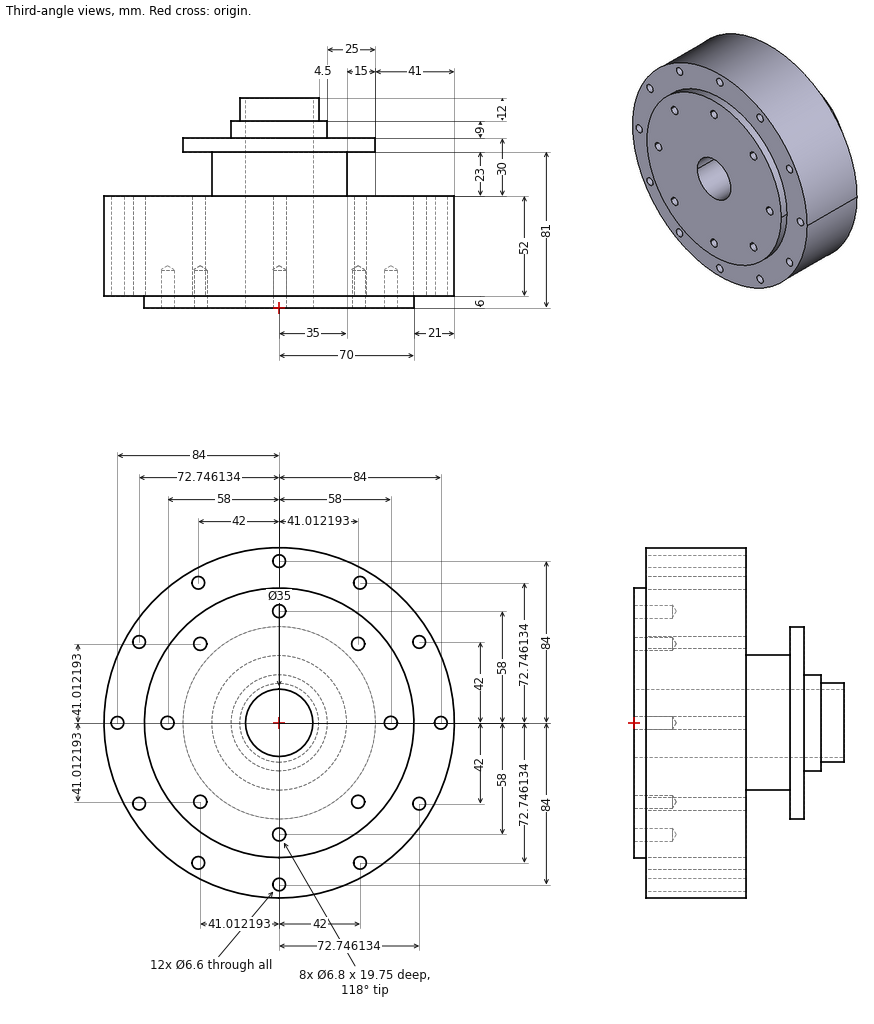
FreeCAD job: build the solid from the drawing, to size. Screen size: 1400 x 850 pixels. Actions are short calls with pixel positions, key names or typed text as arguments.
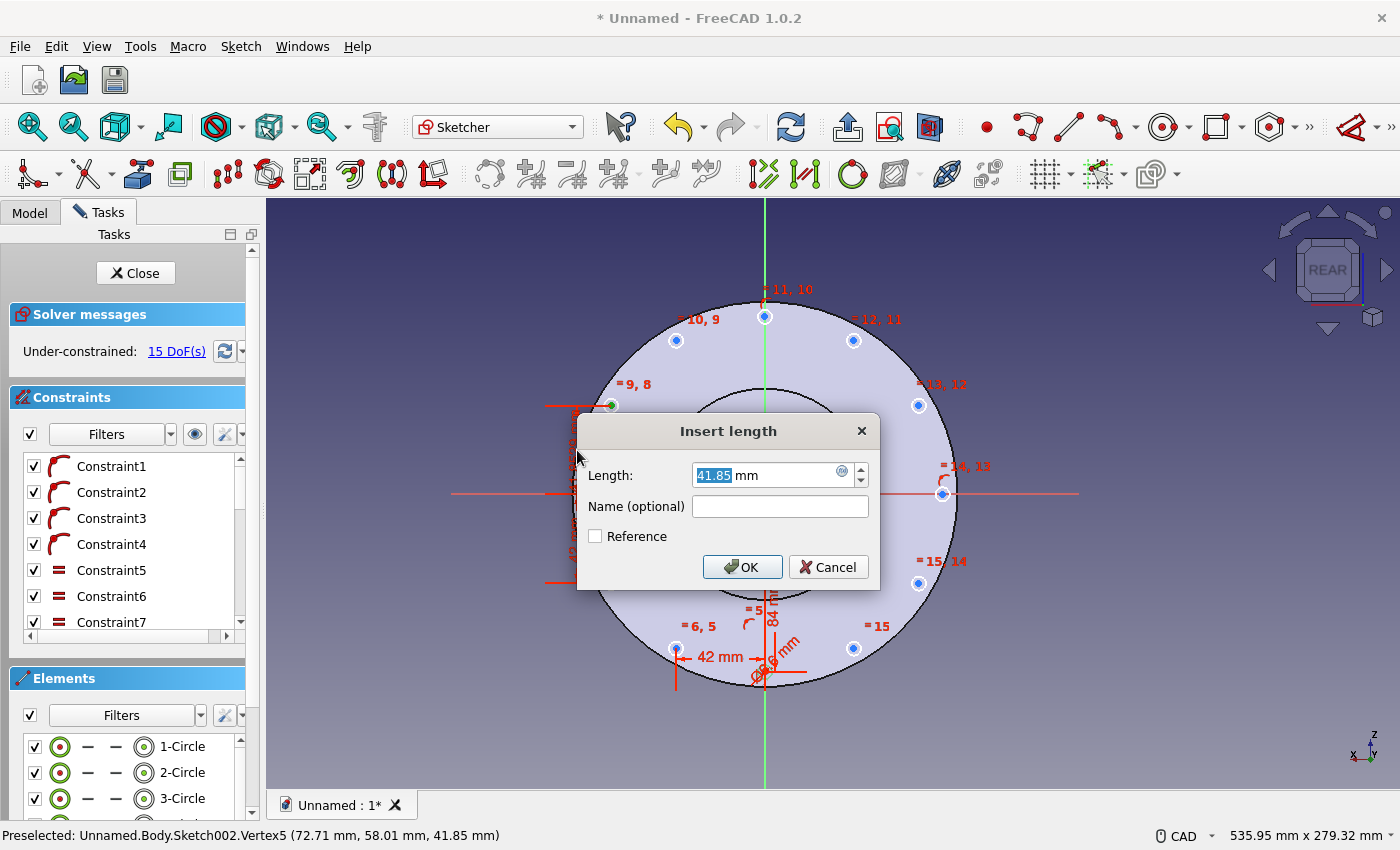
text(42)
key(Return)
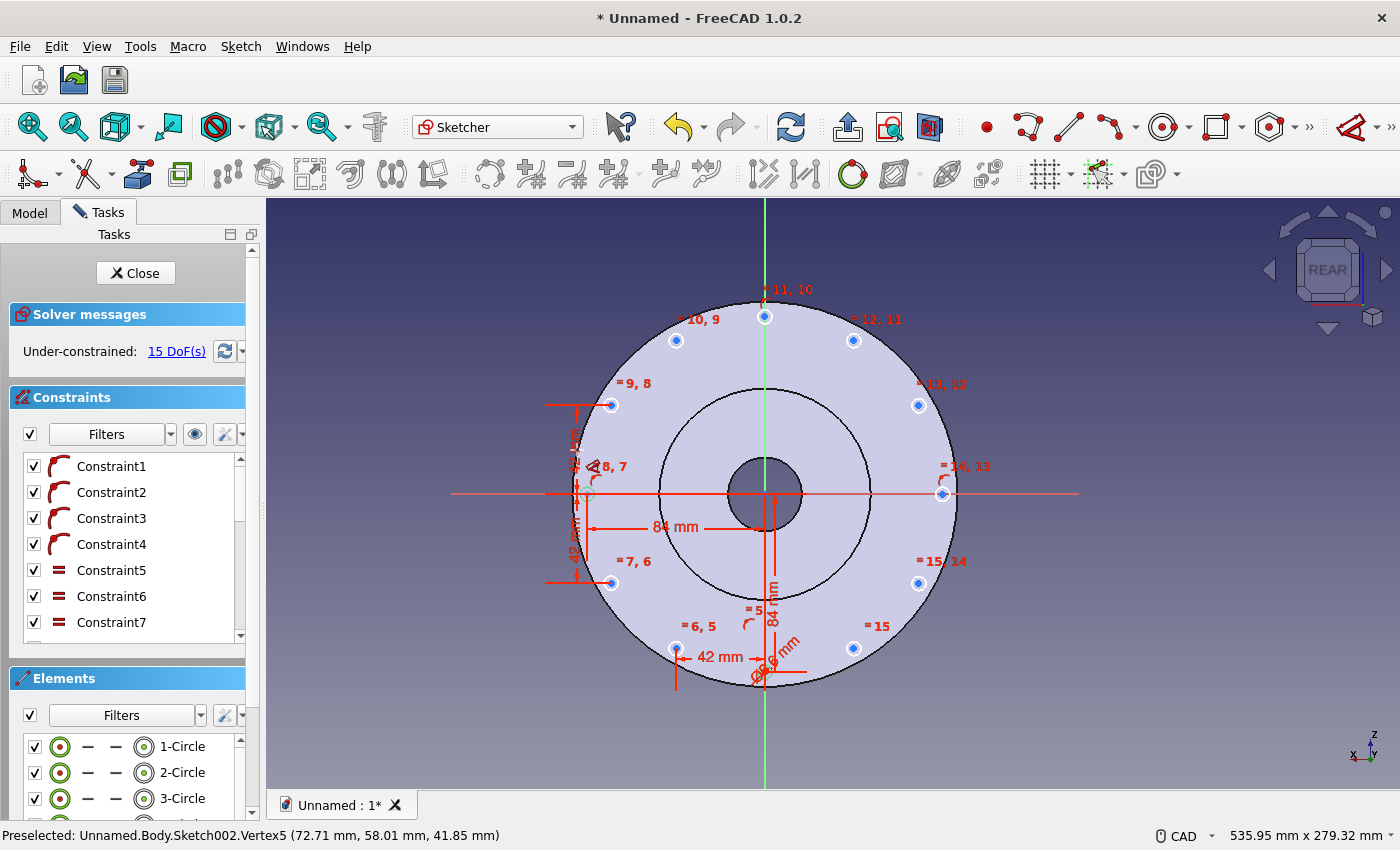
click(676, 341)
click(721, 307)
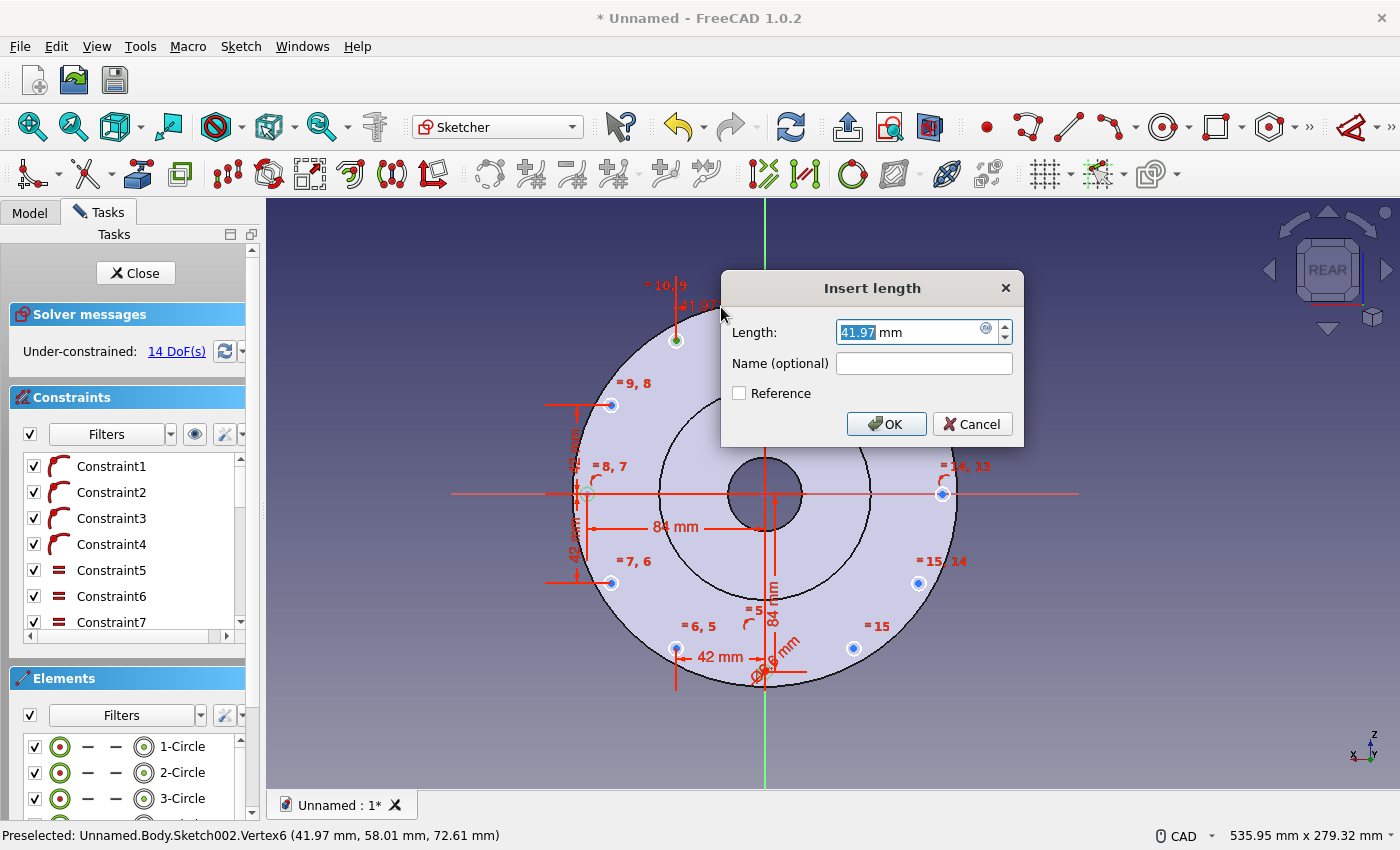
text(42)
key(Return)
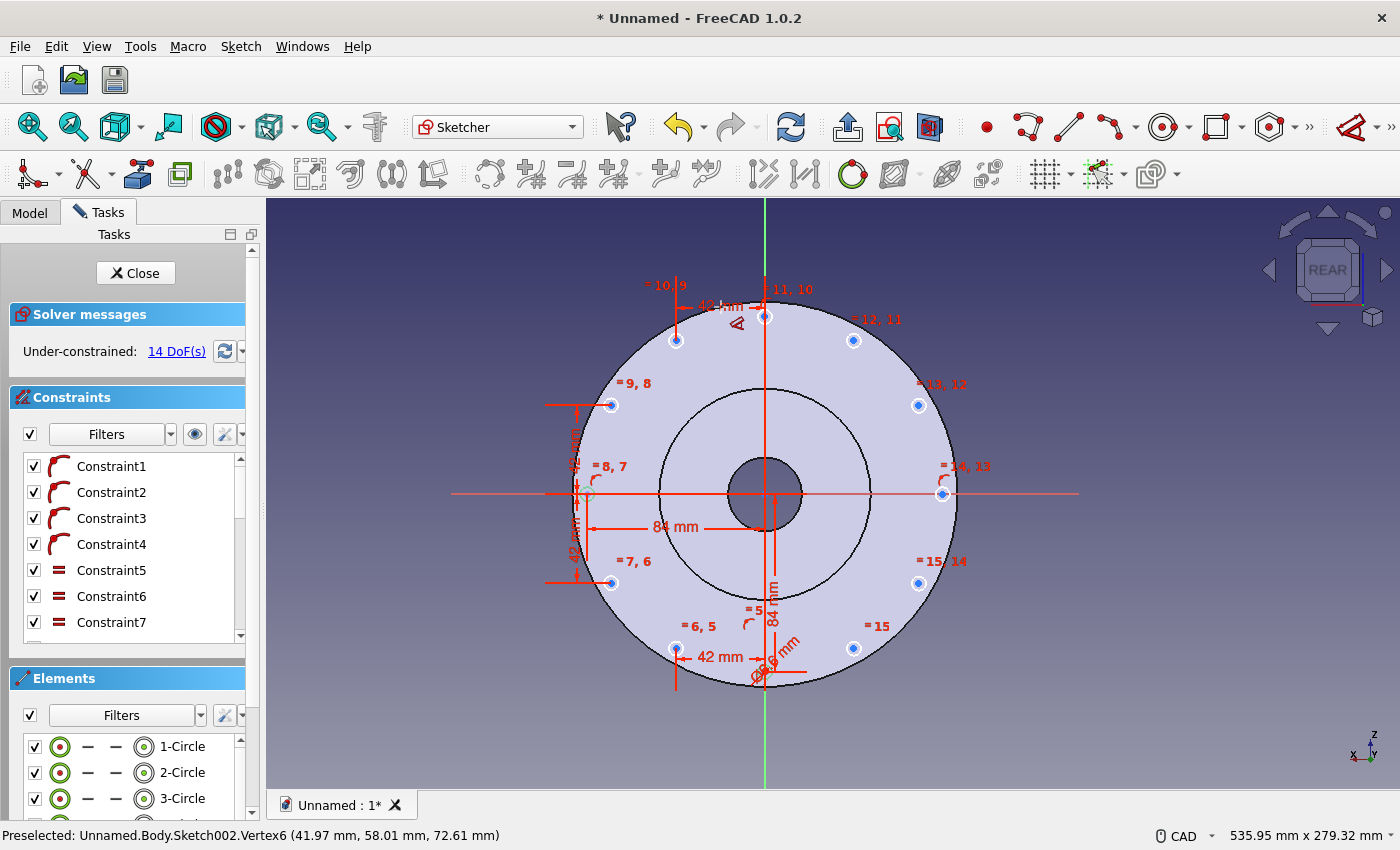
click(765, 317)
click(799, 406)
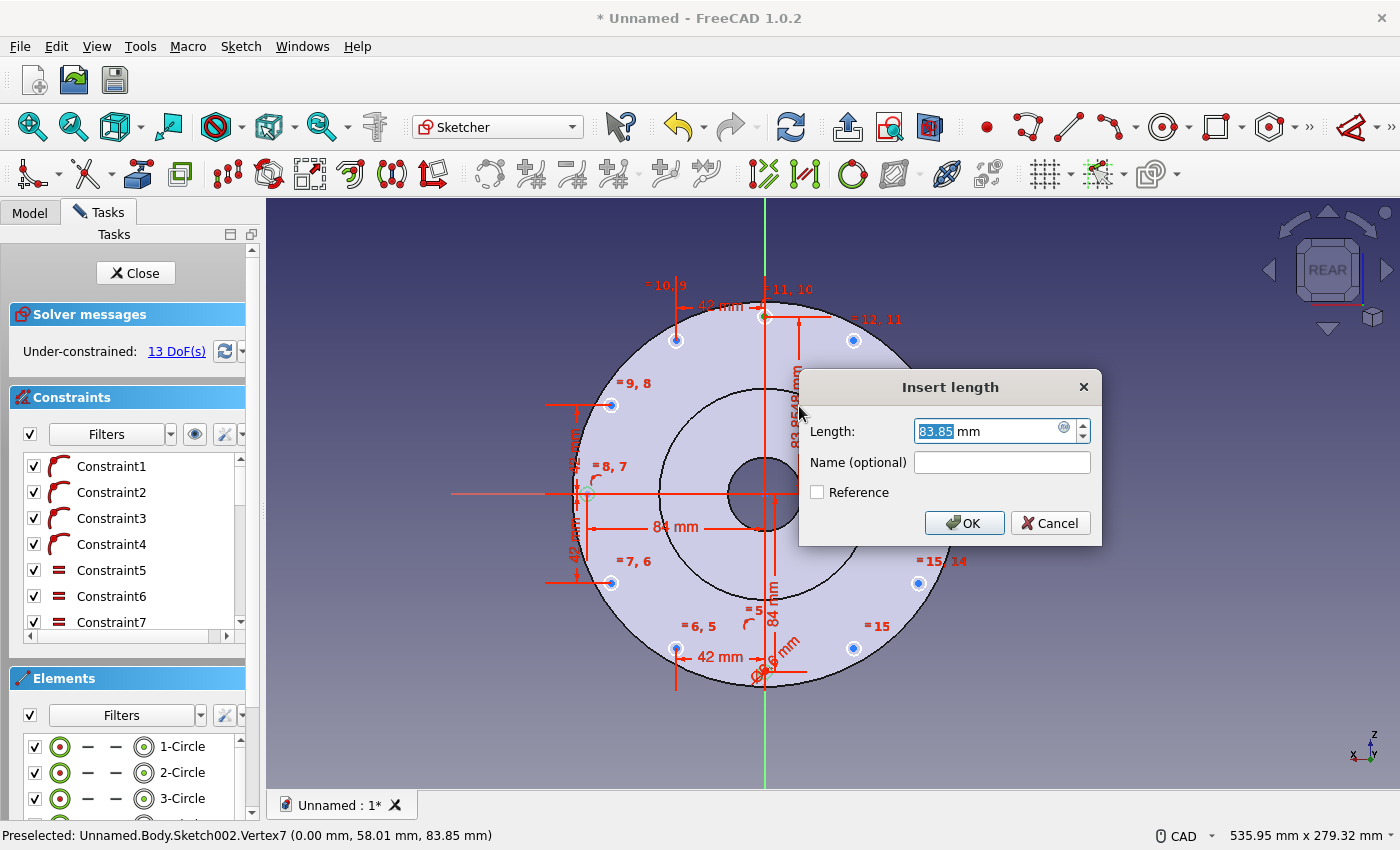
text(84)
key(Return)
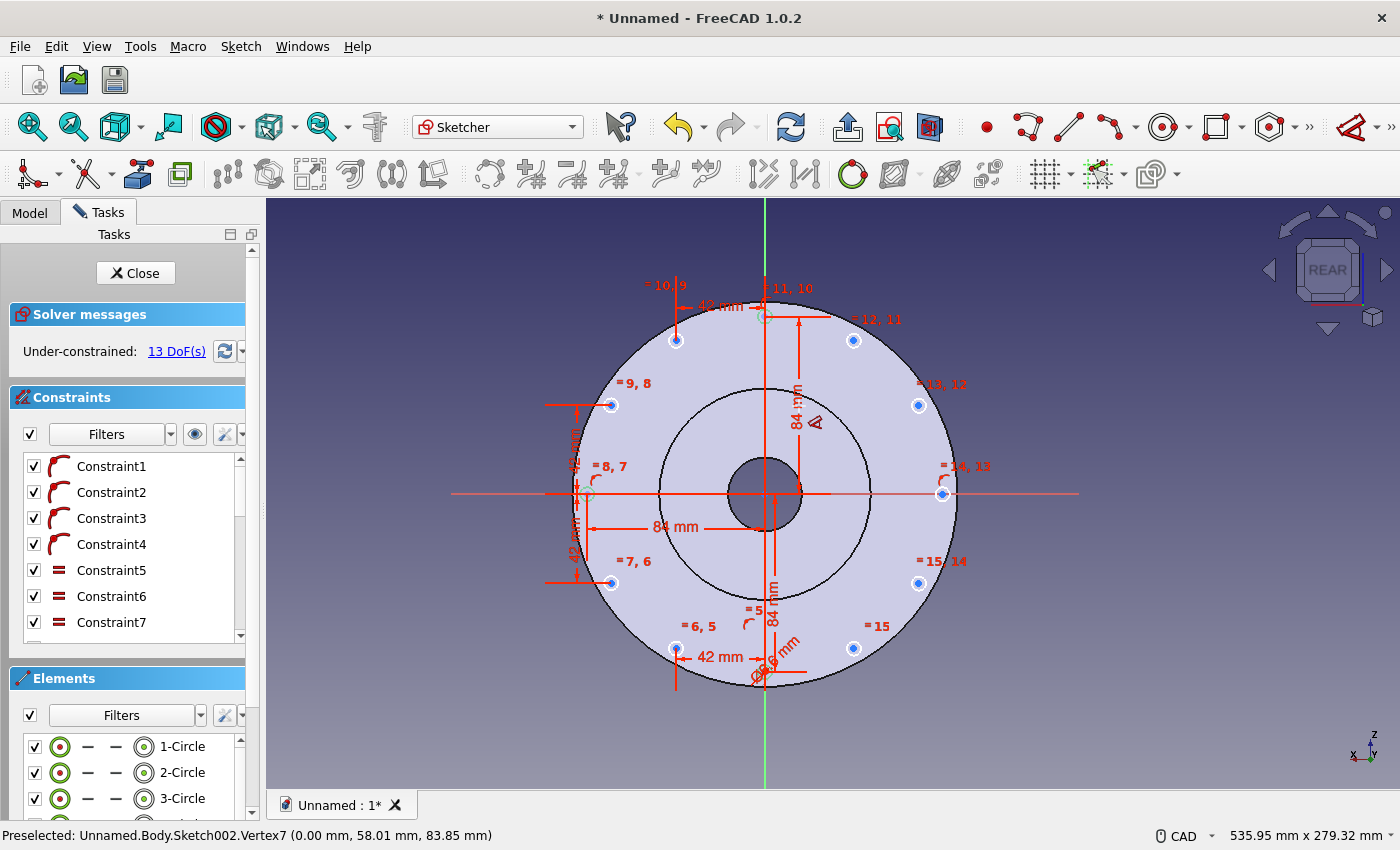
click(854, 341)
click(809, 307)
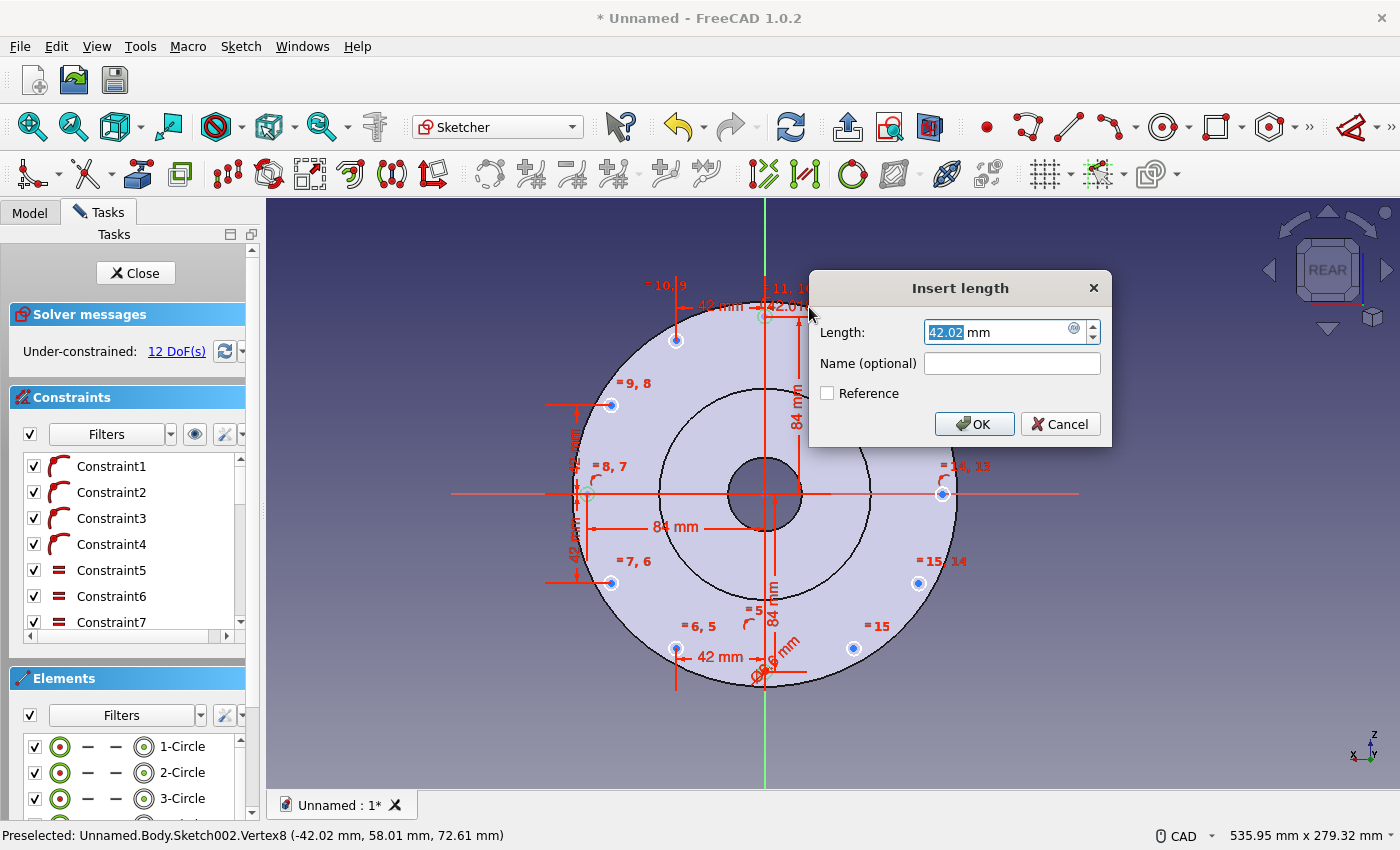
text(42)
key(Return)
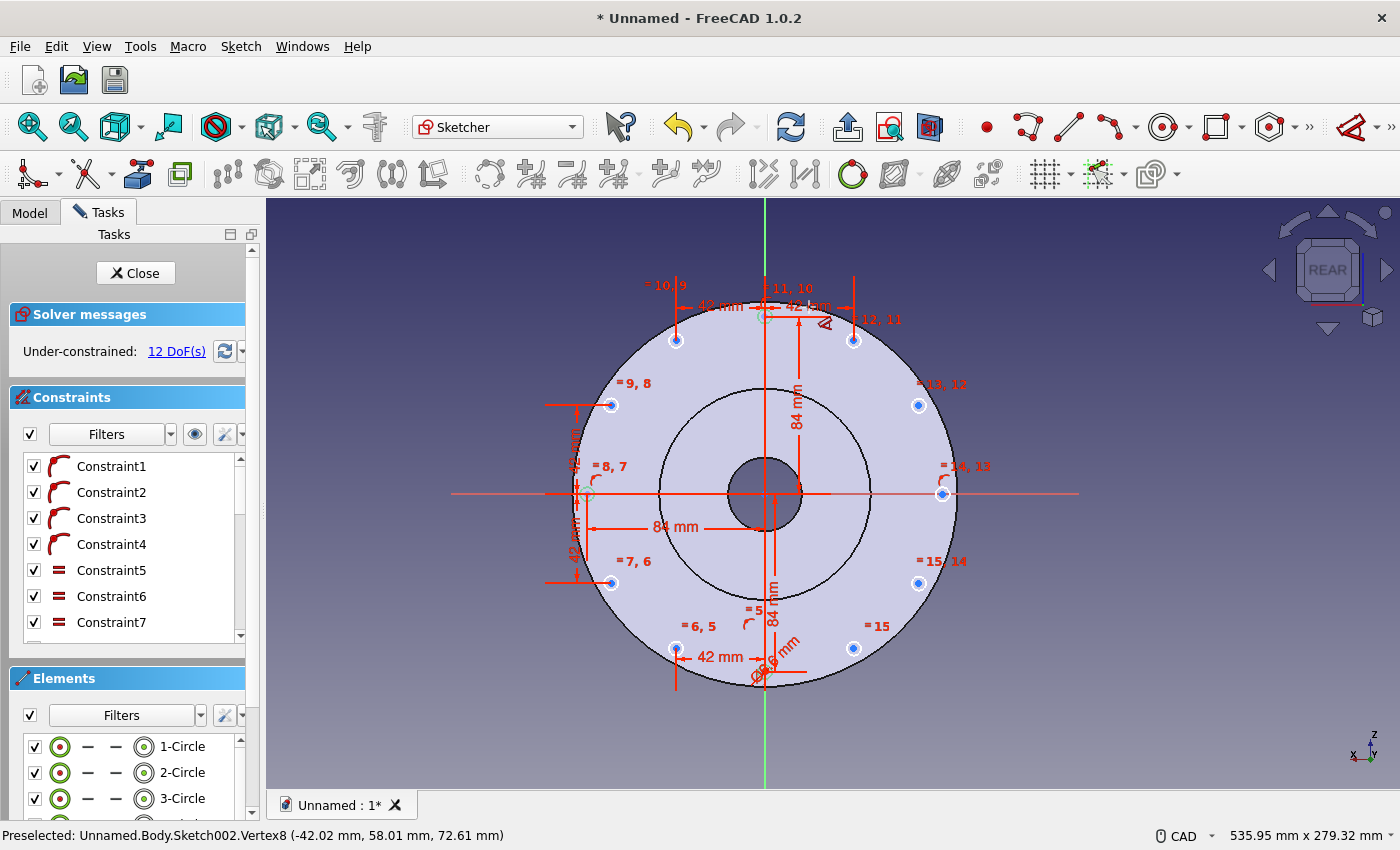
click(919, 406)
click(953, 450)